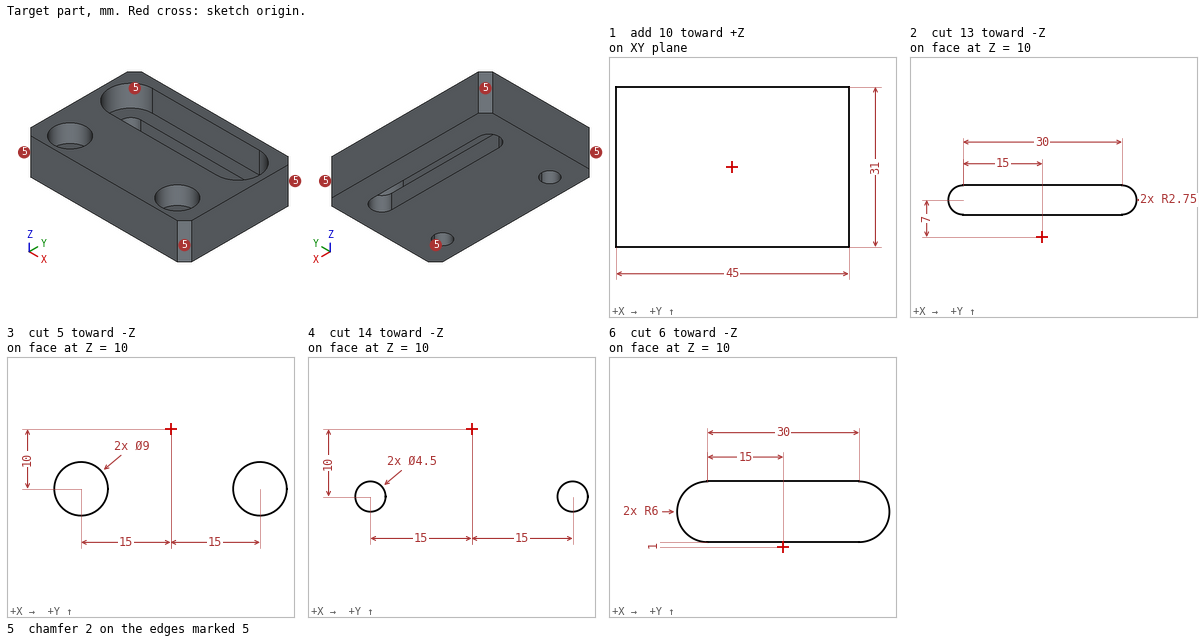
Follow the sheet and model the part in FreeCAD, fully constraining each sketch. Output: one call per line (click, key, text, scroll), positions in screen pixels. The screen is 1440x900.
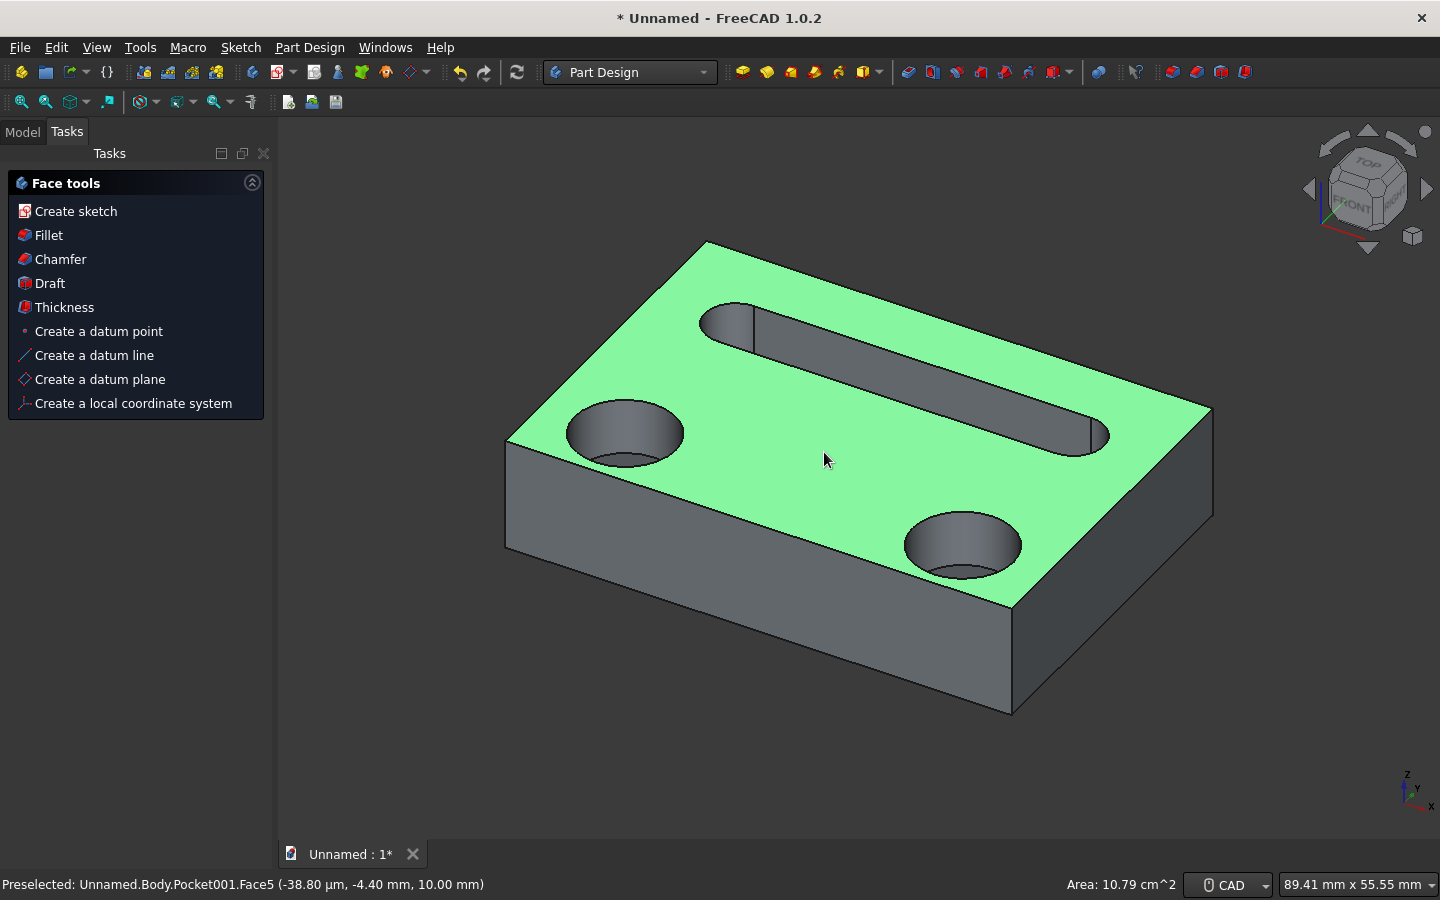
click(278, 72)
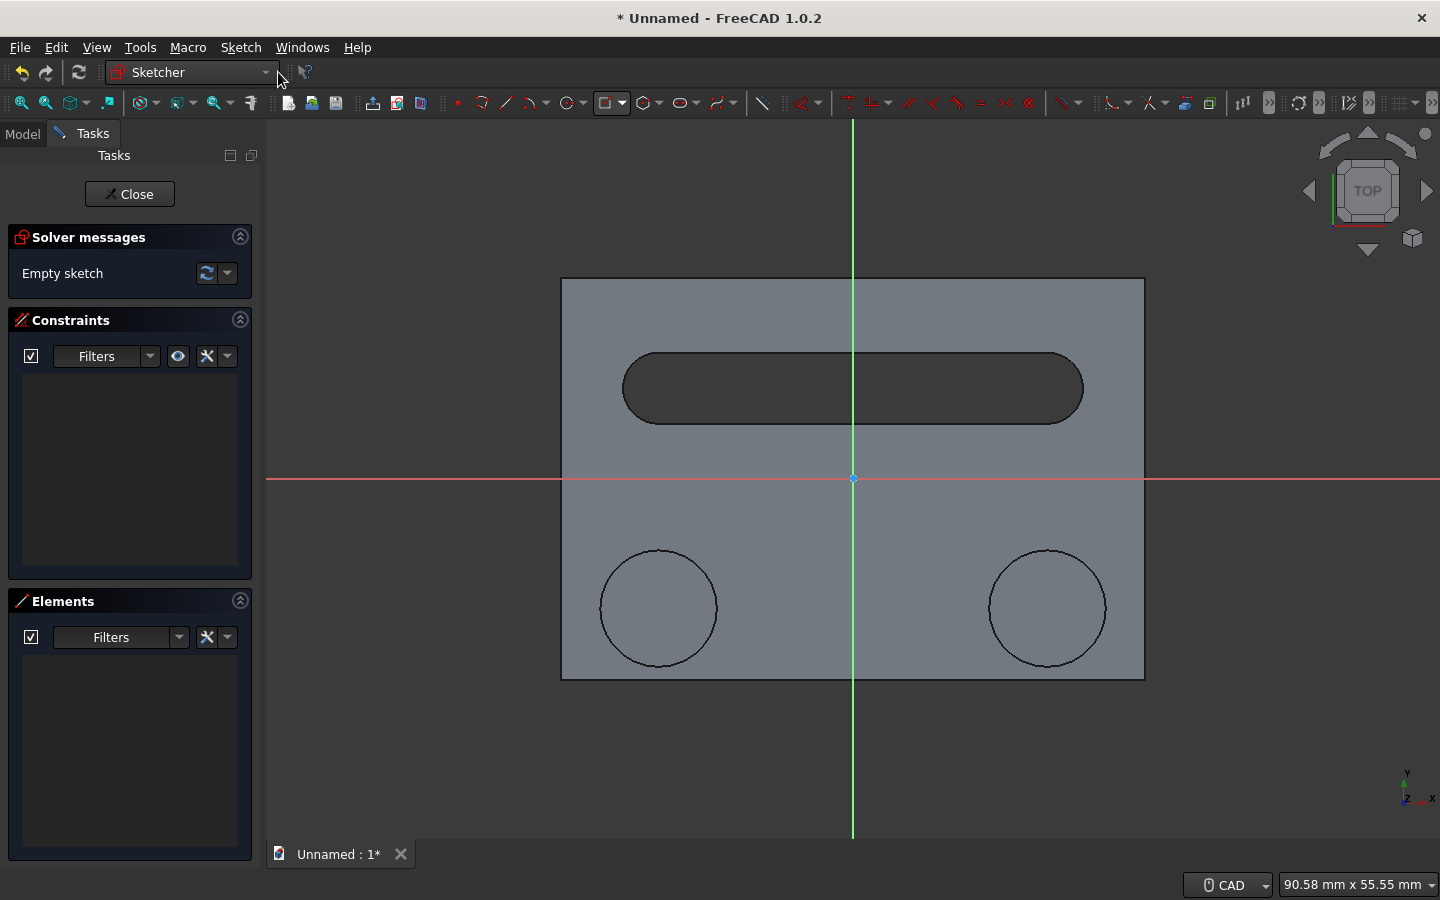
scroll(992, 720, up, 2)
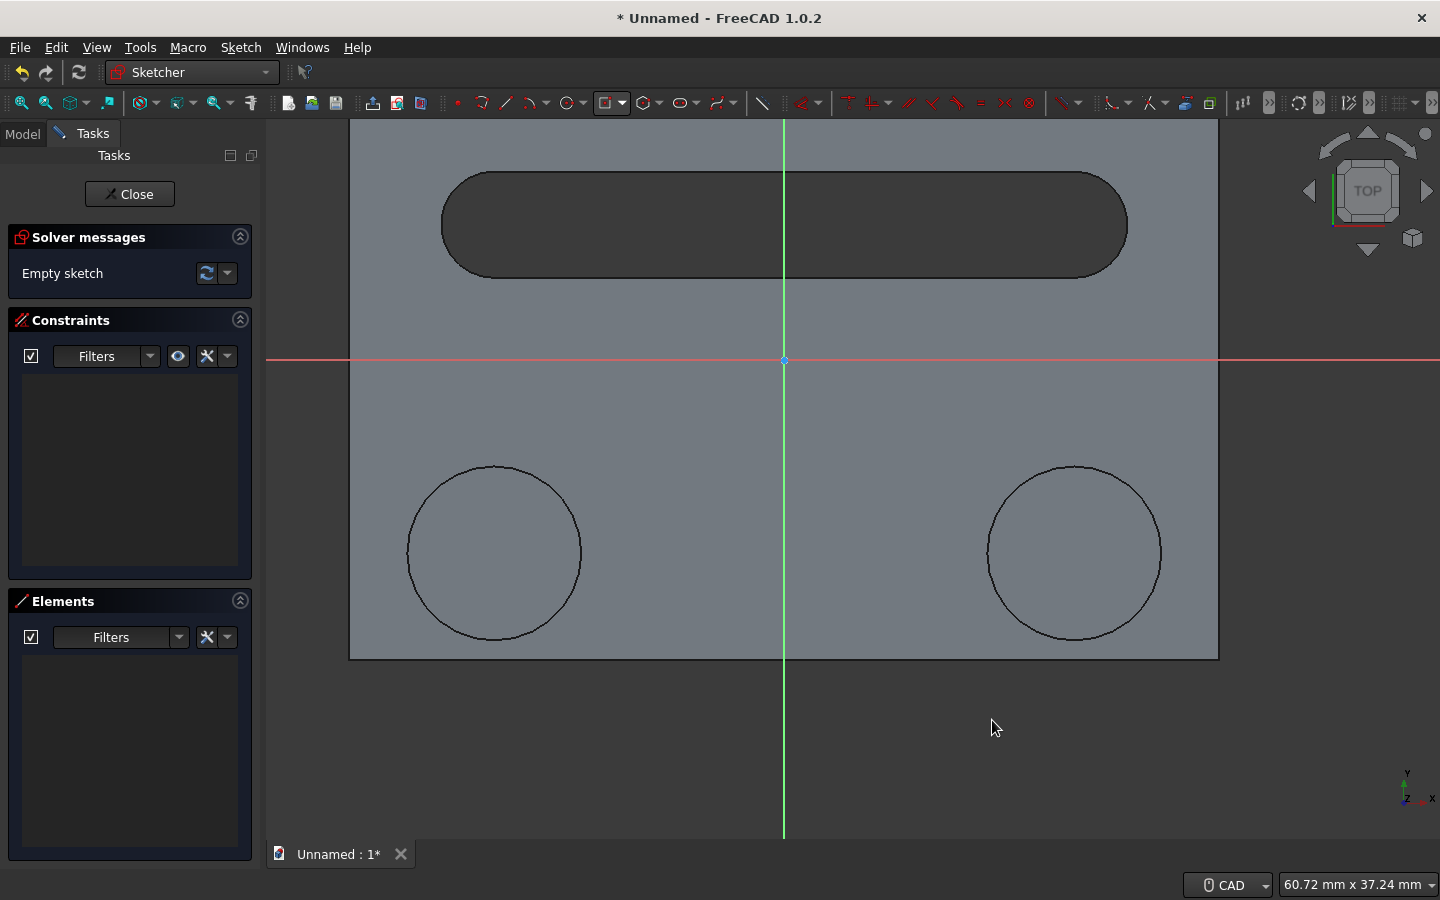
click(568, 104)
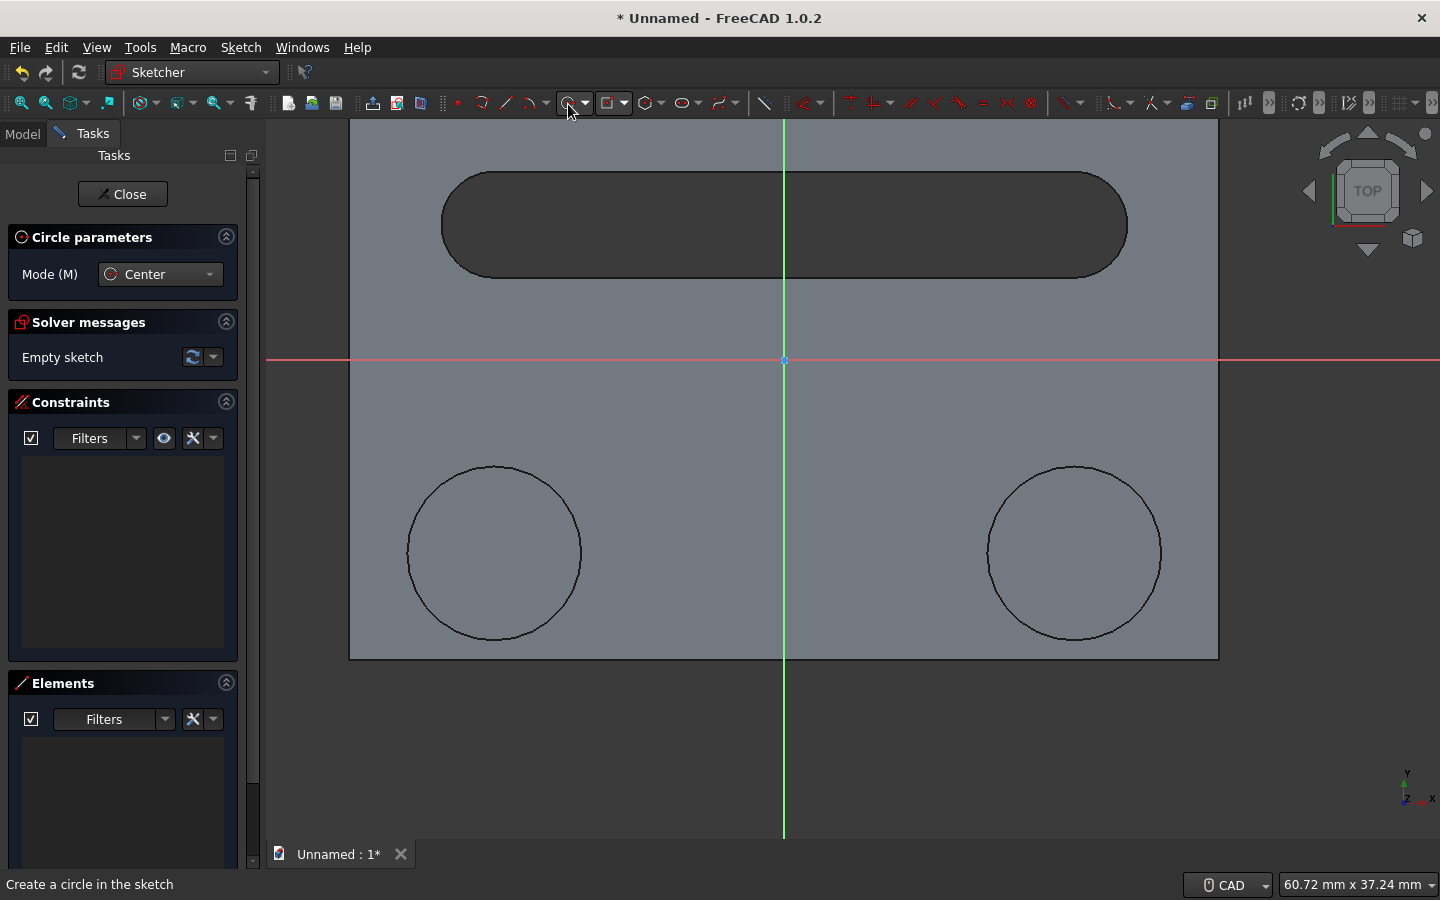
click(494, 553)
click(525, 523)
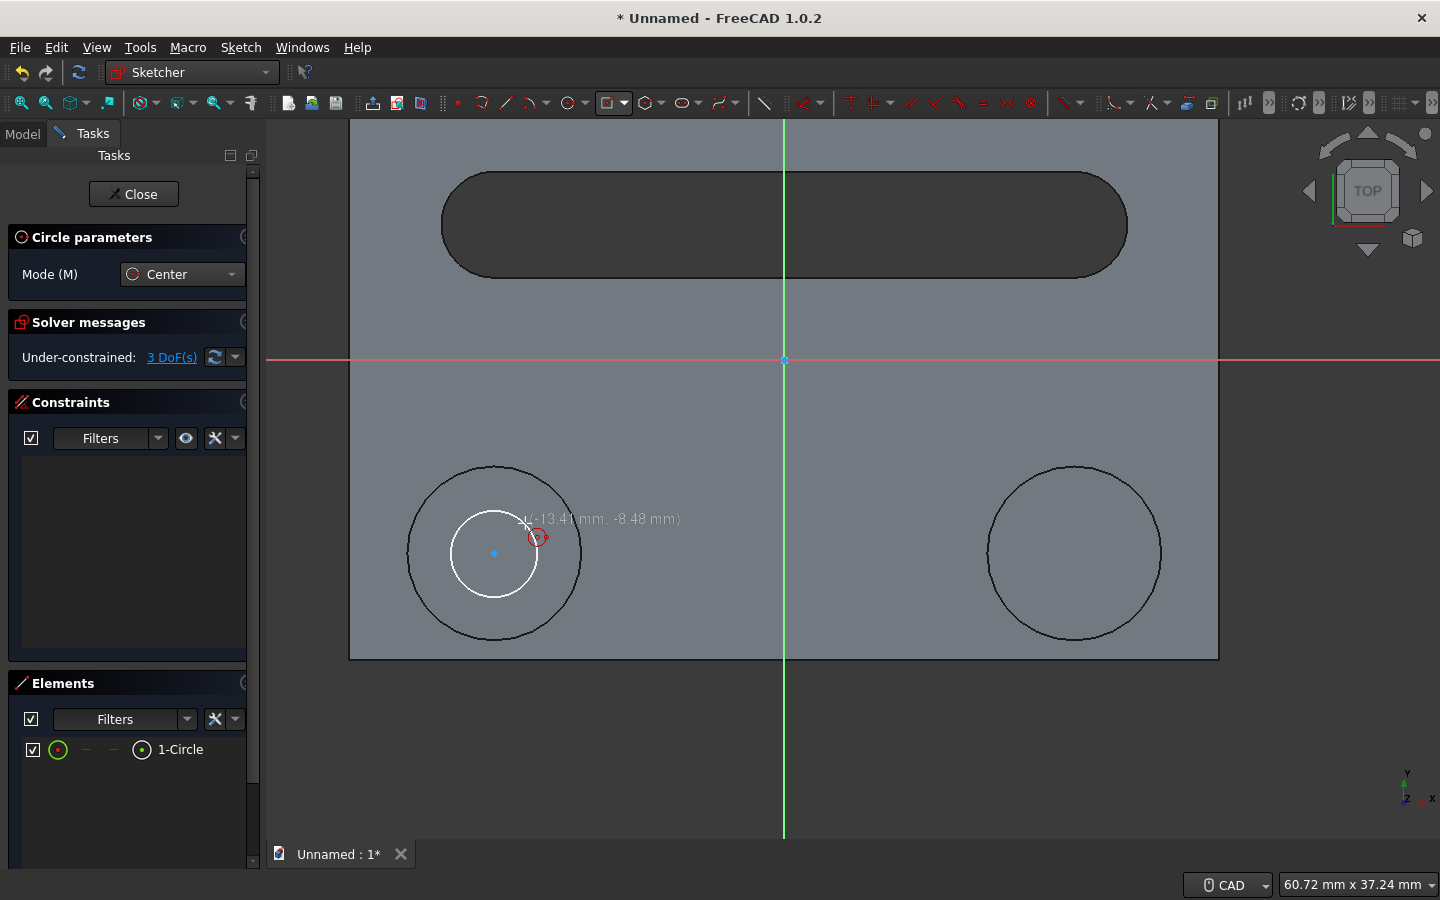
click(1074, 553)
click(1105, 523)
key(Escape)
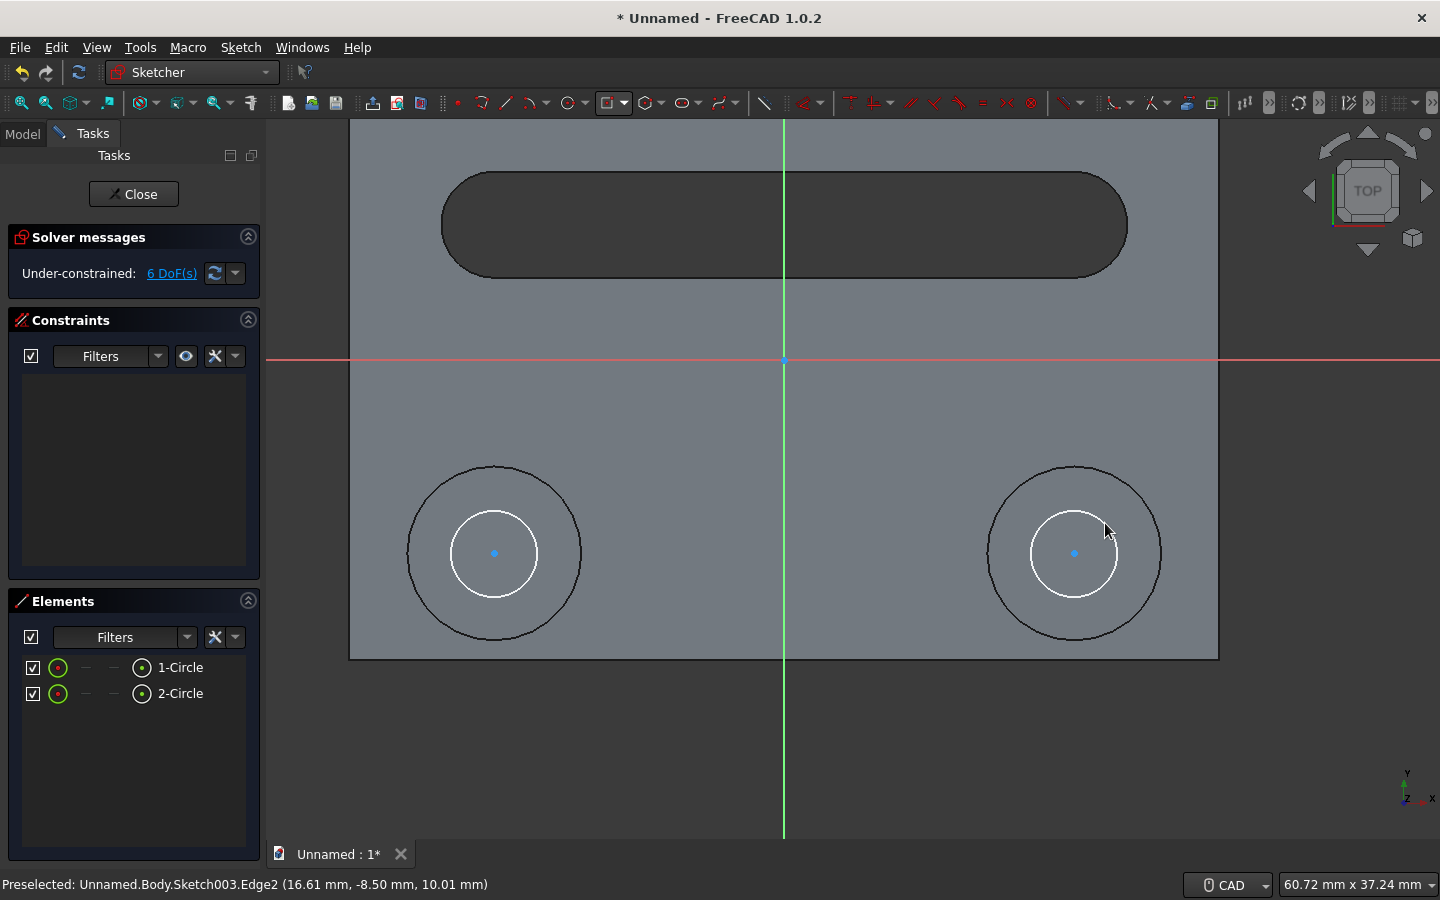
click(524, 523)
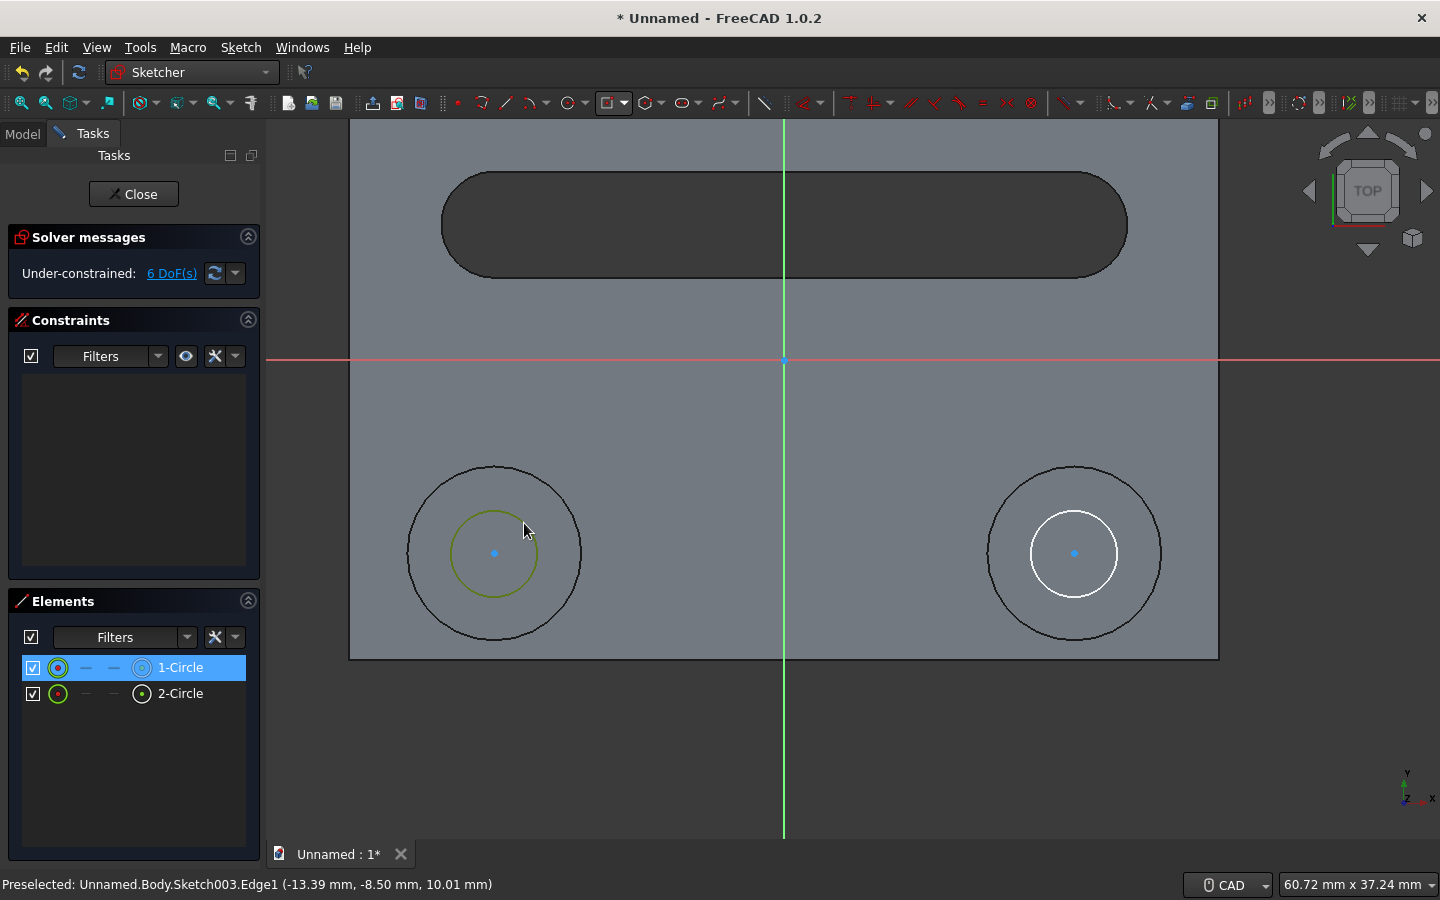
click(1104, 523)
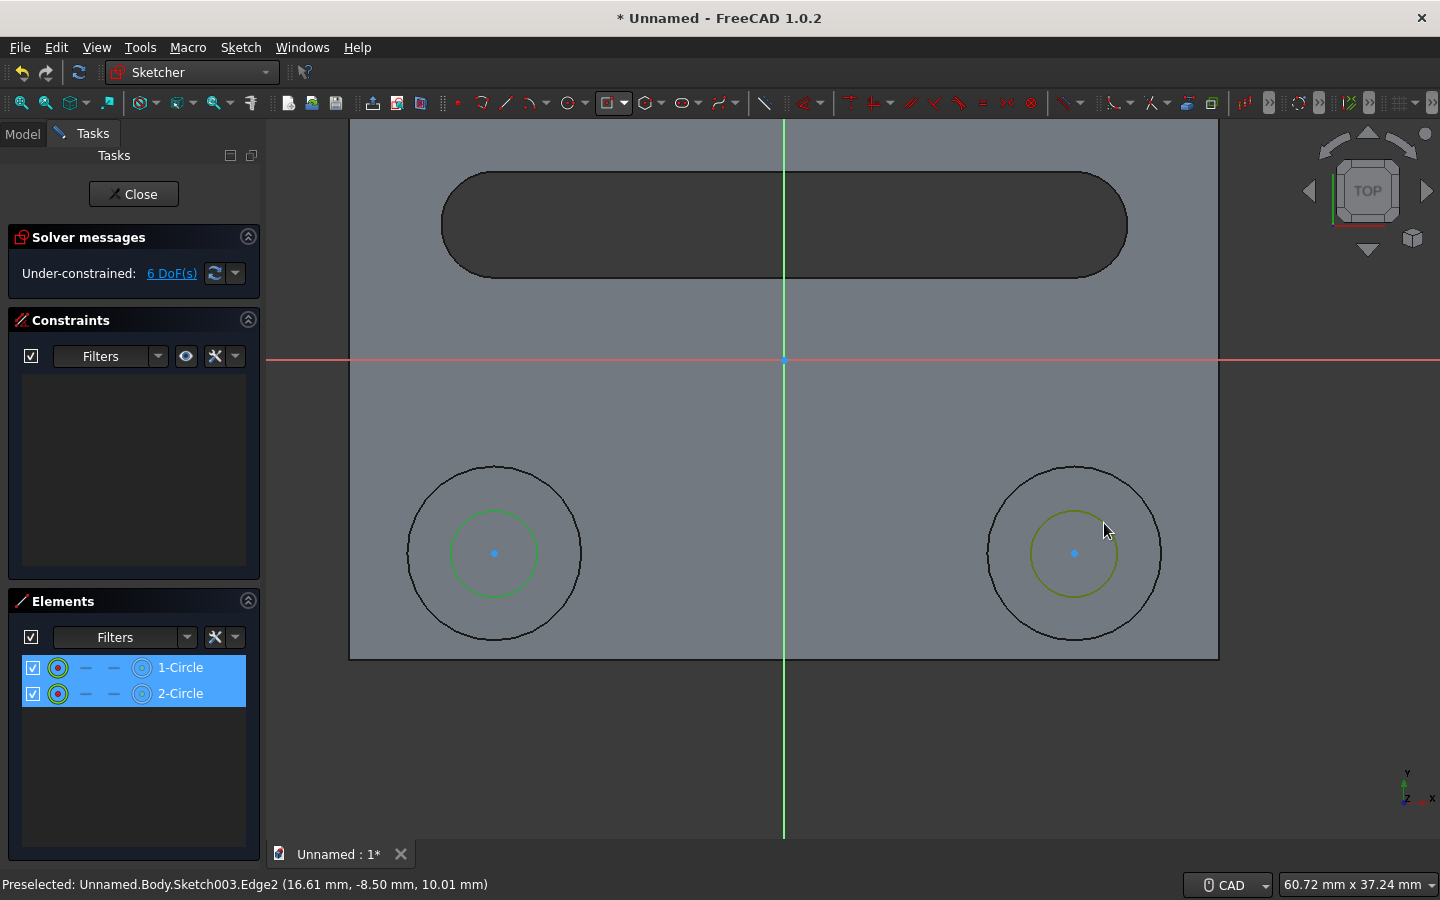
click(984, 104)